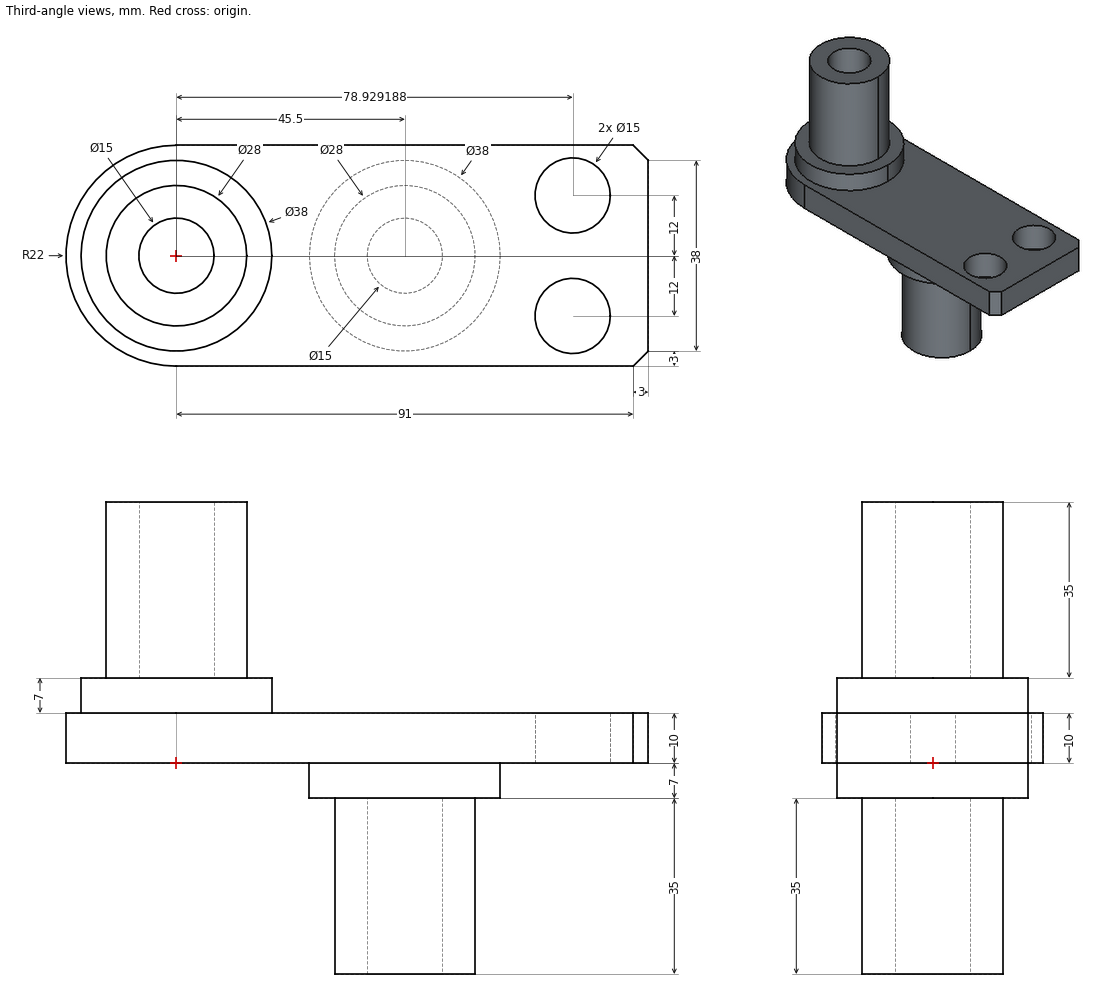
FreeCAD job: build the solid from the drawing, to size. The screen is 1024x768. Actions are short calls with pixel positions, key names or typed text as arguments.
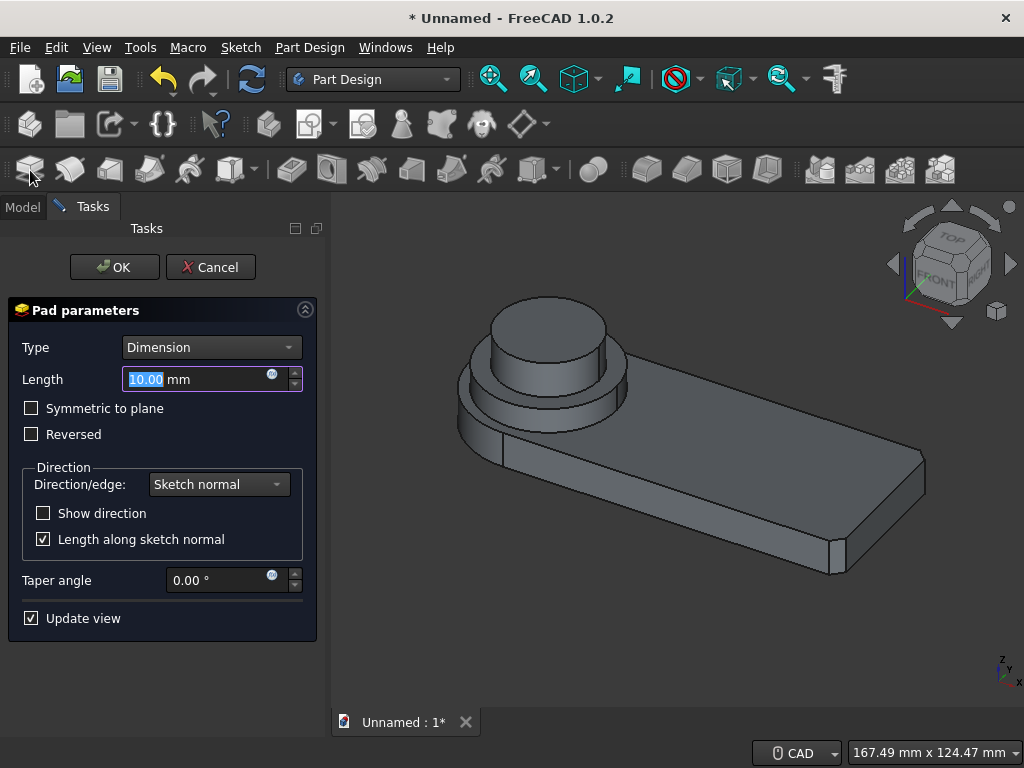
text(35)
key(Tab)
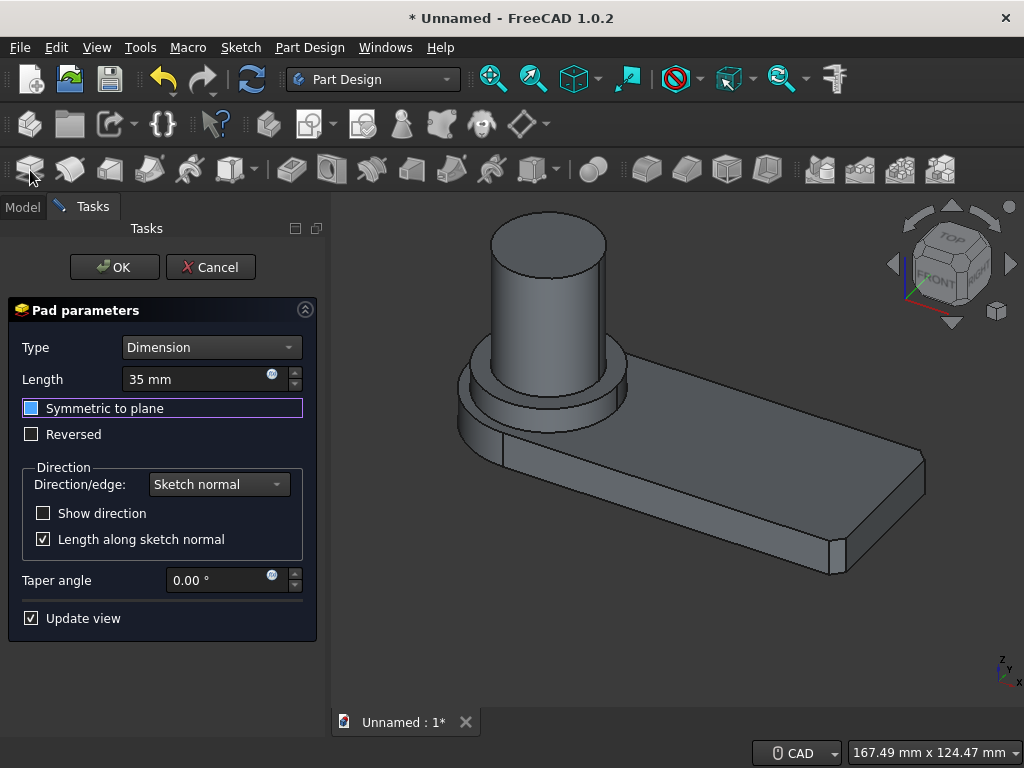
click(115, 267)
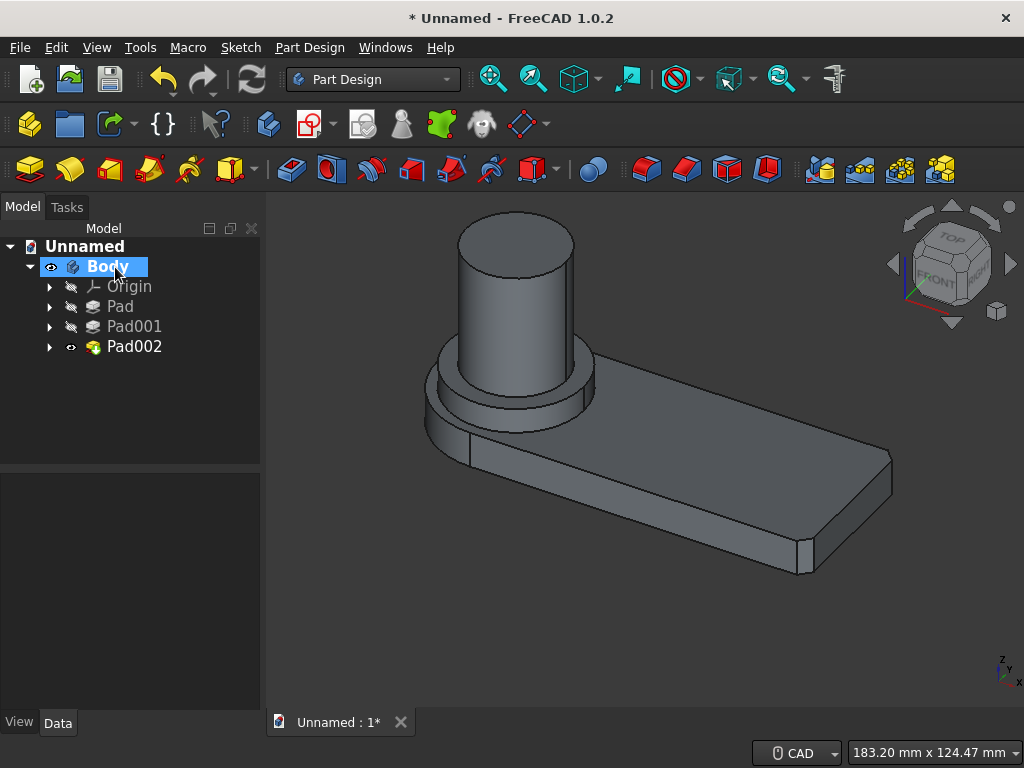
click(494, 80)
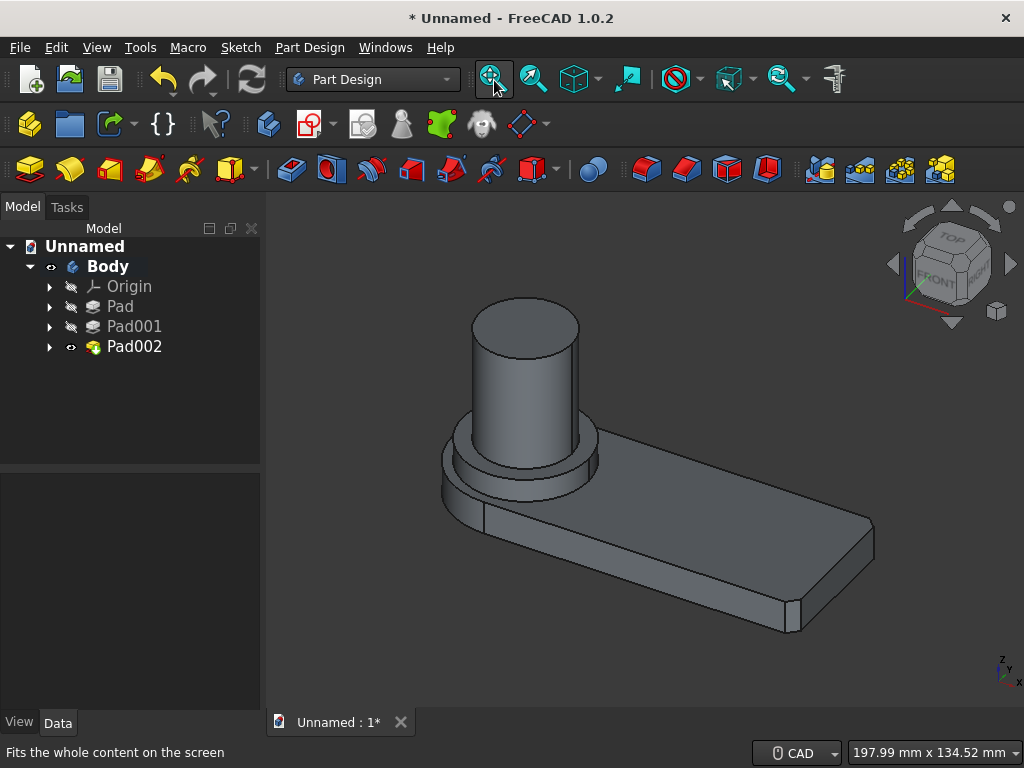
key(5)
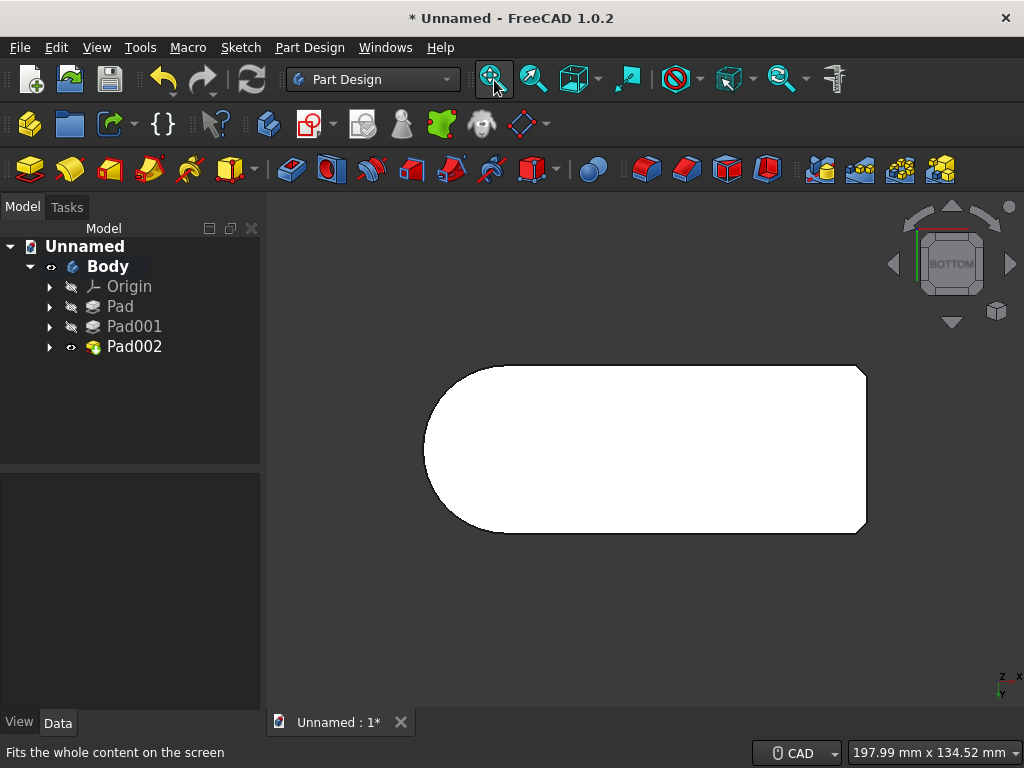
click(772, 448)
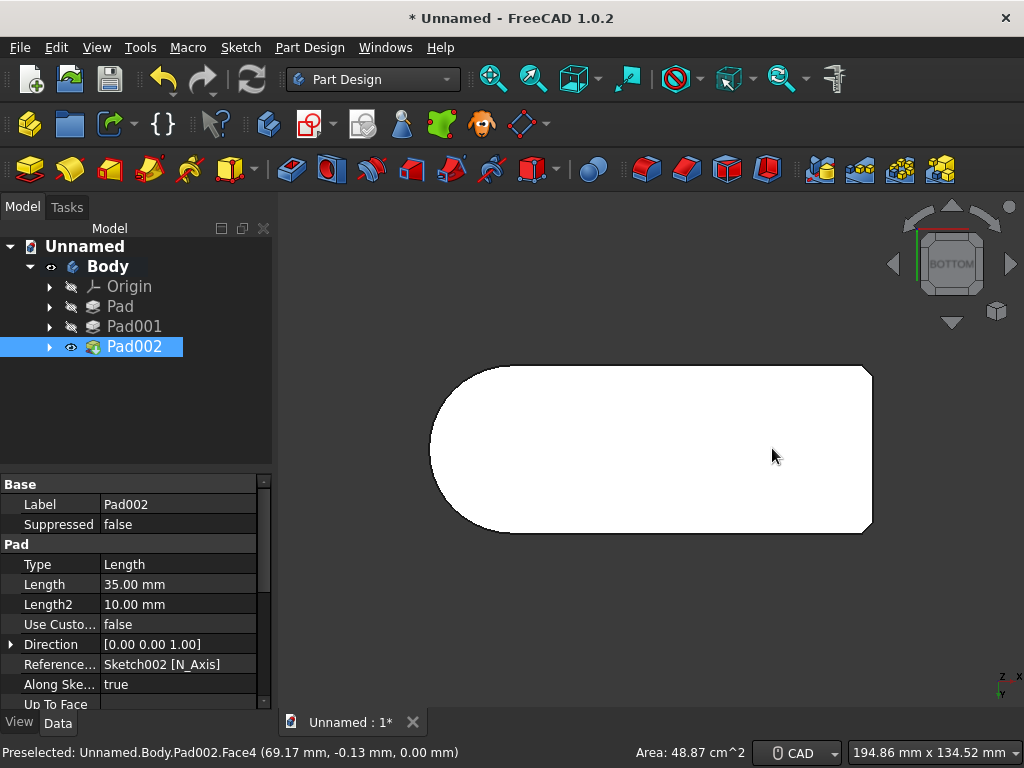
click(310, 124)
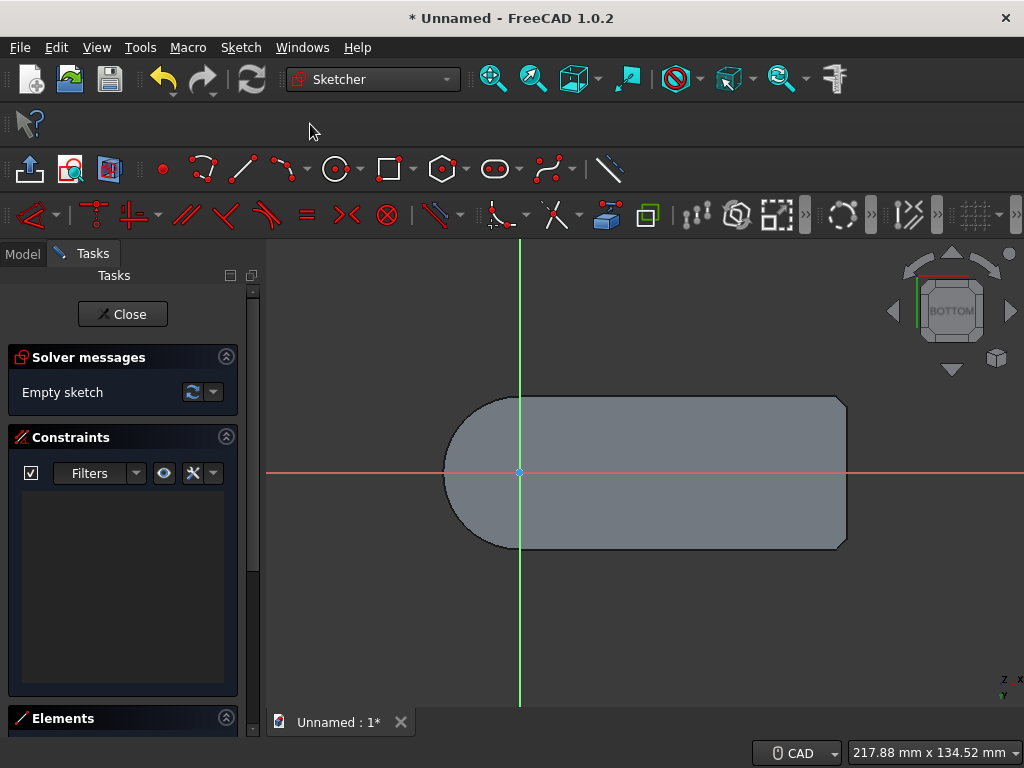
scroll(699, 473, up, 3)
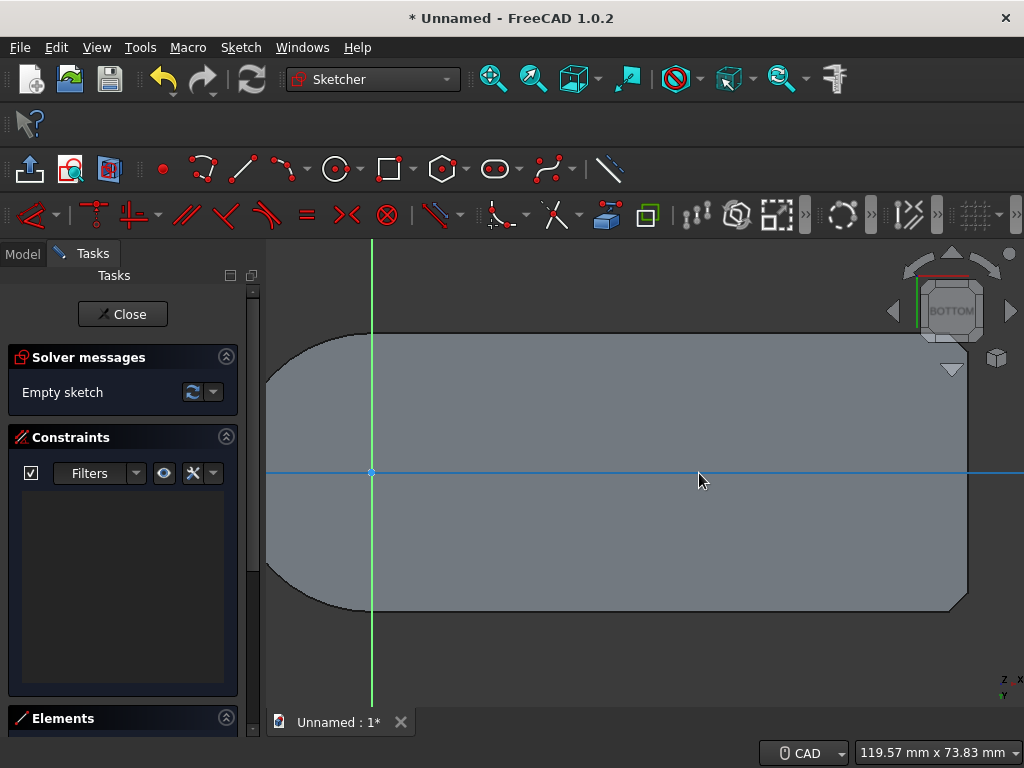
click(336, 170)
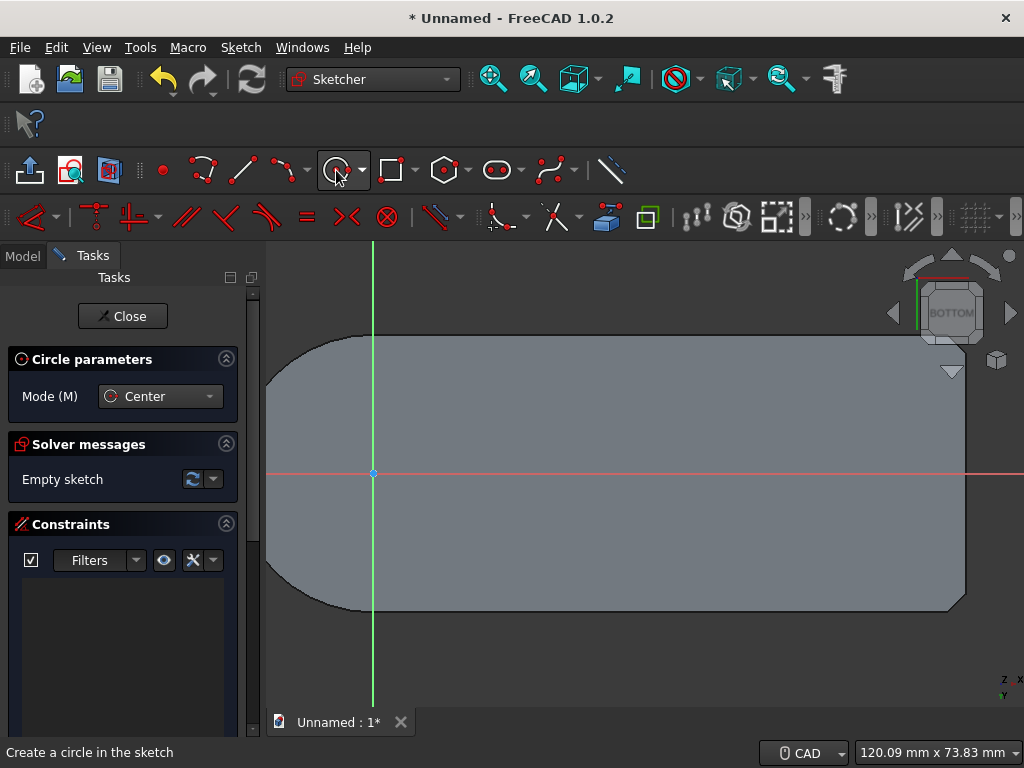
click(660, 474)
move(745, 389)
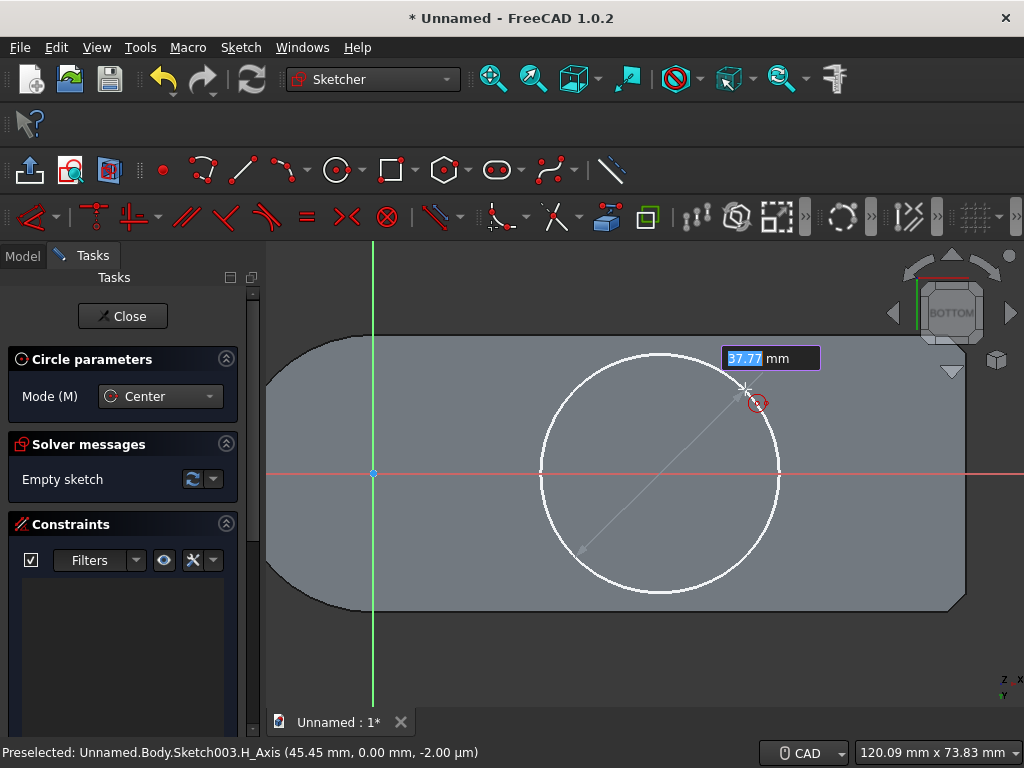
text(38)
key(Return)
key(Escape)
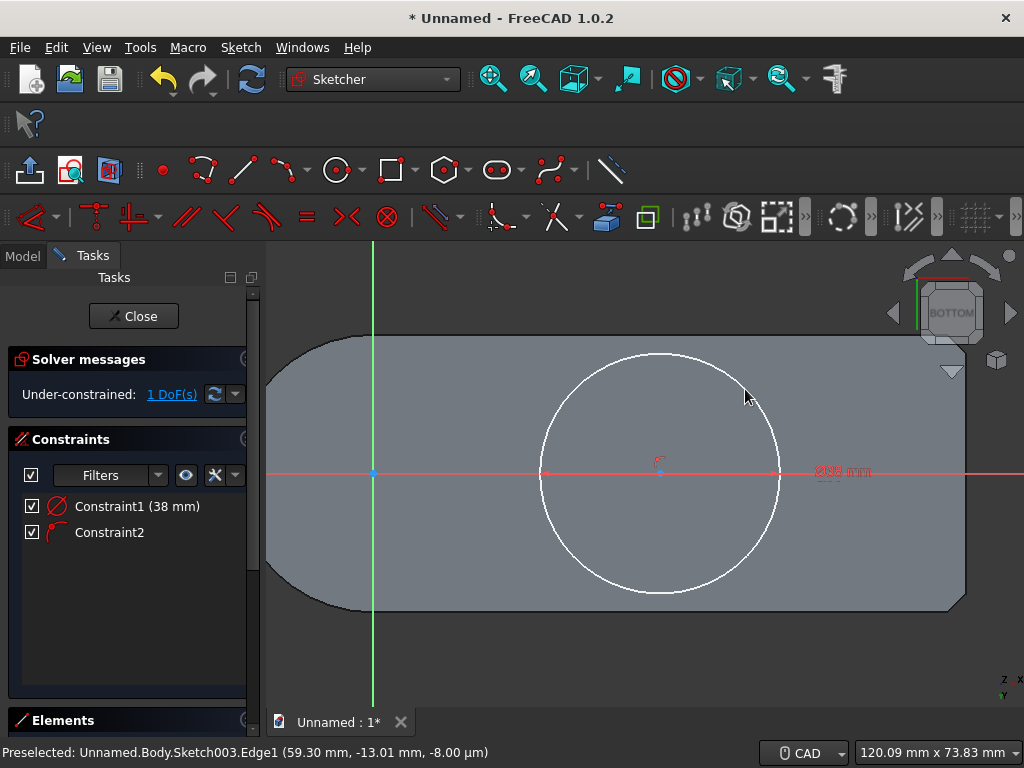
click(32, 218)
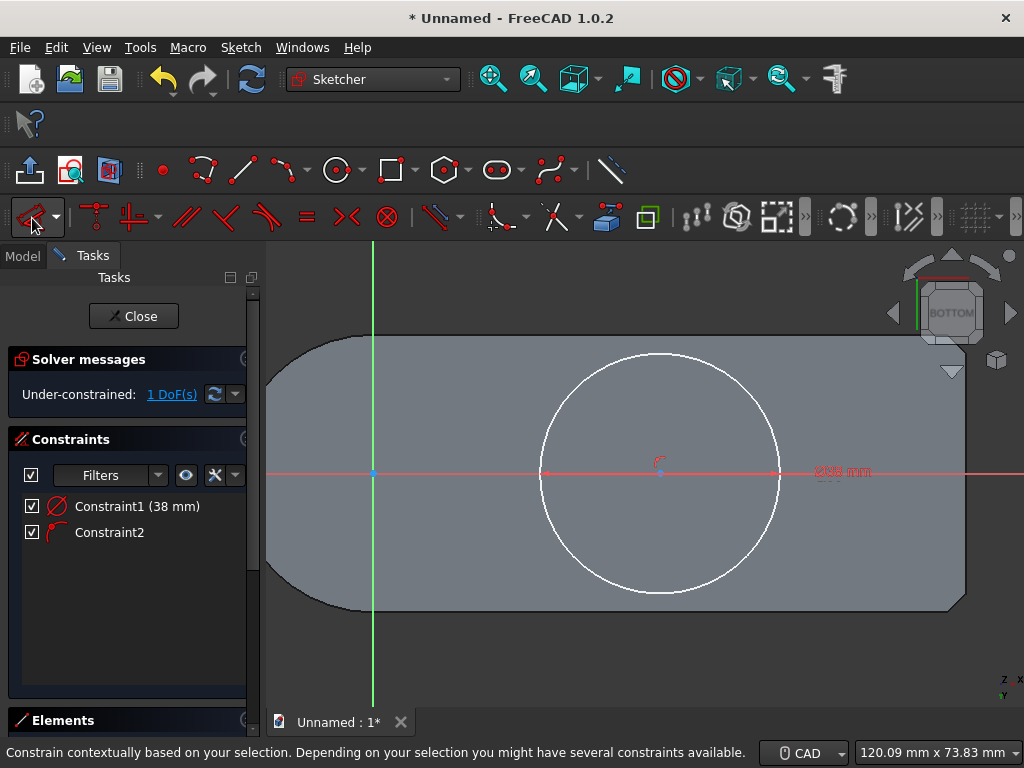
click(660, 474)
click(517, 508)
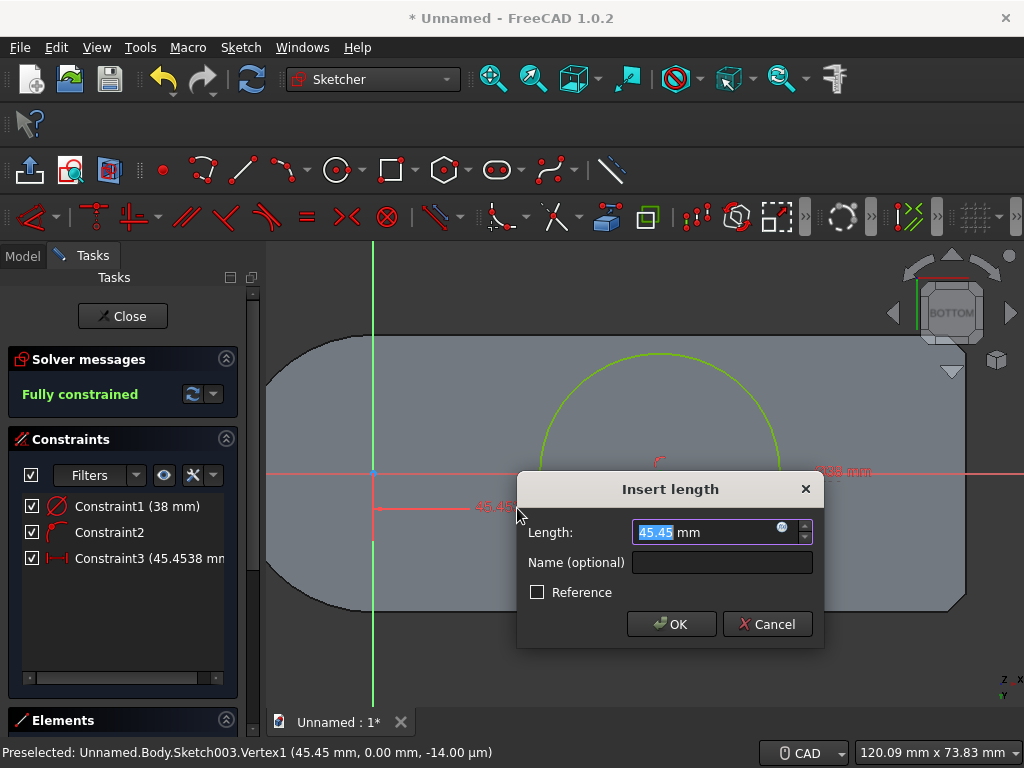
text(45.5)
key(Return)
key(Escape)